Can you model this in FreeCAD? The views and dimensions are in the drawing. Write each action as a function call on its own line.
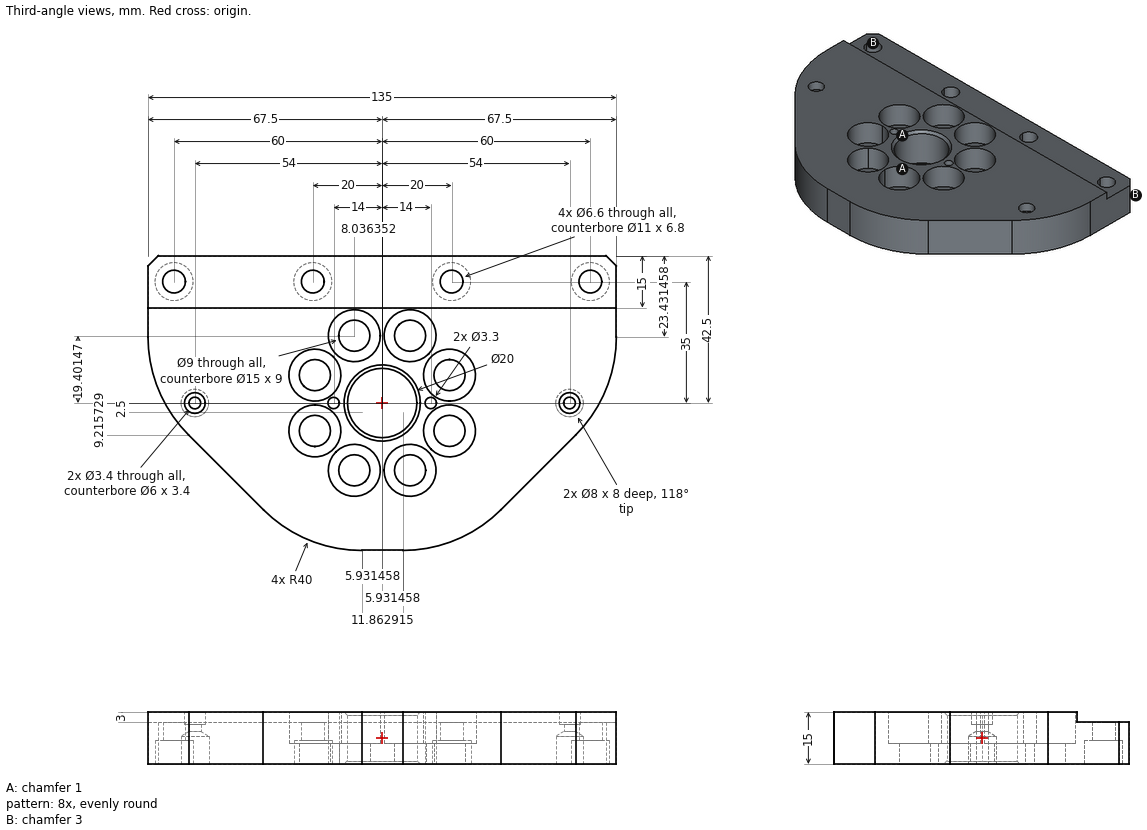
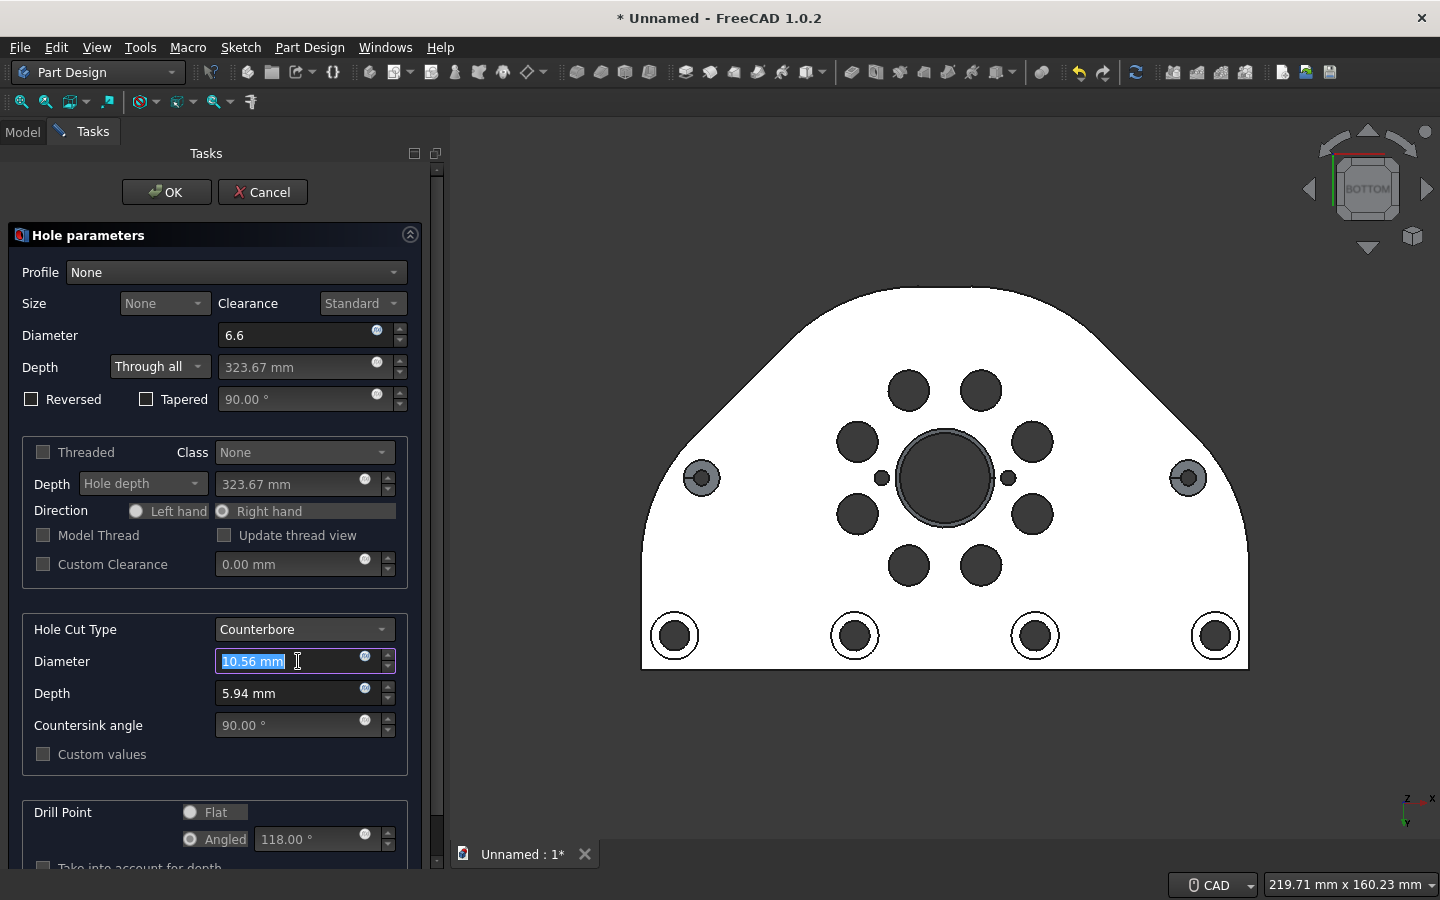
text(11)
key(Tab)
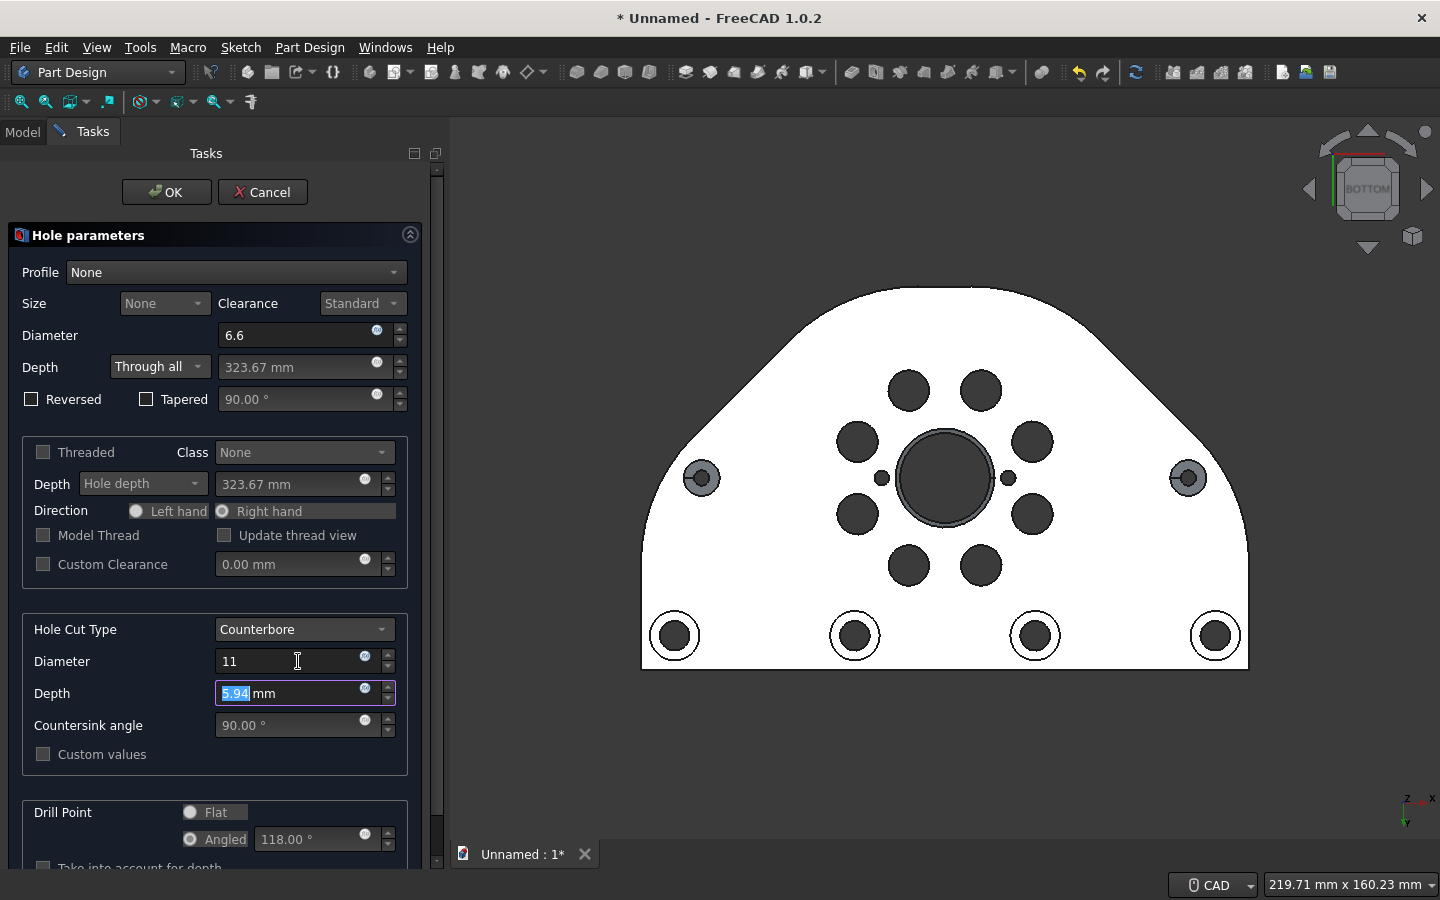
text(6.8)
key(Tab)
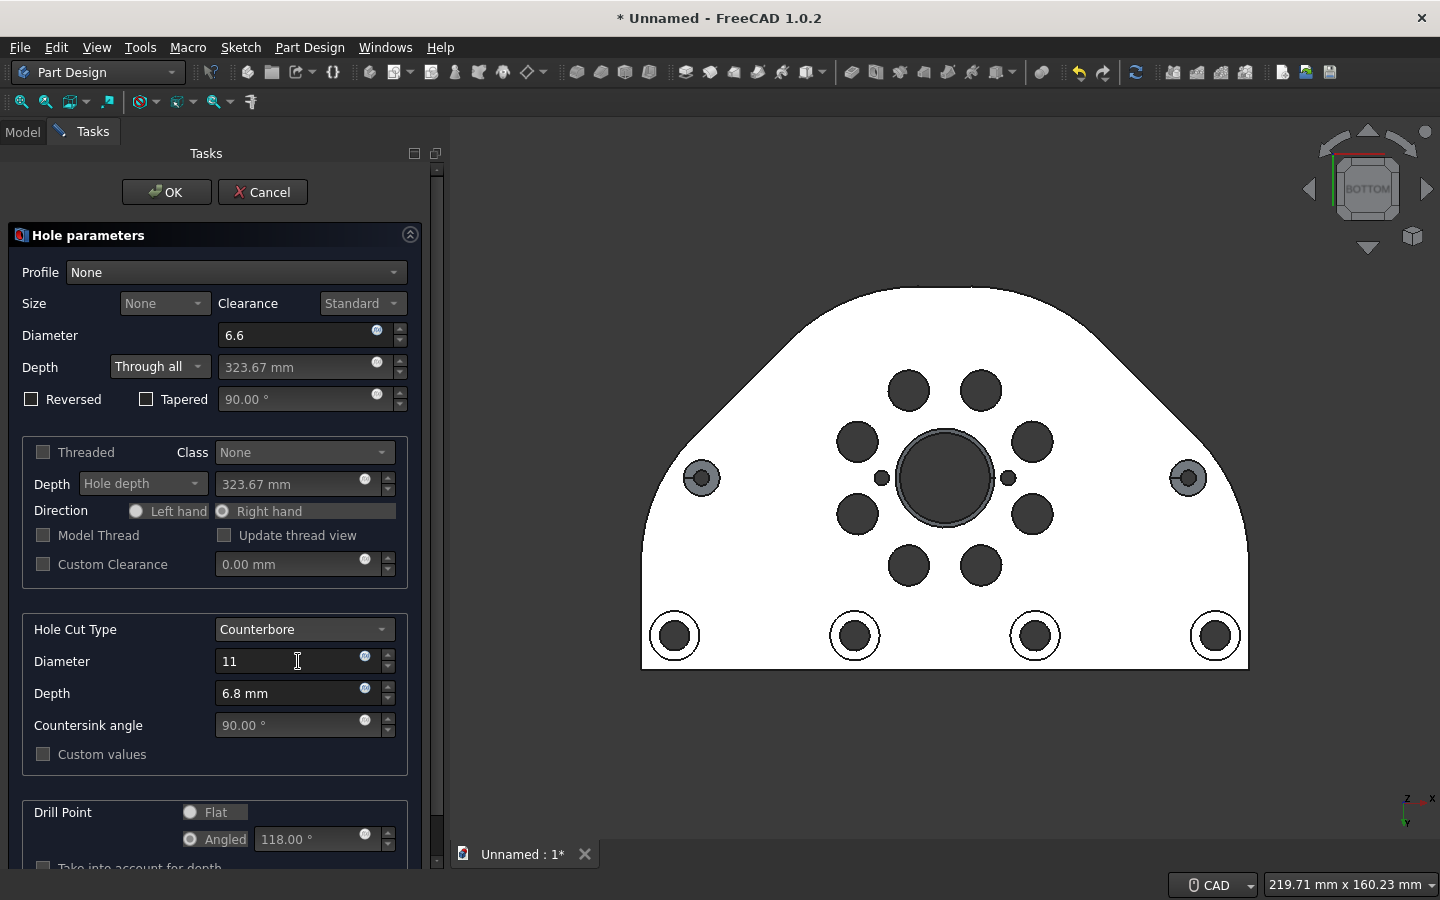
click(167, 192)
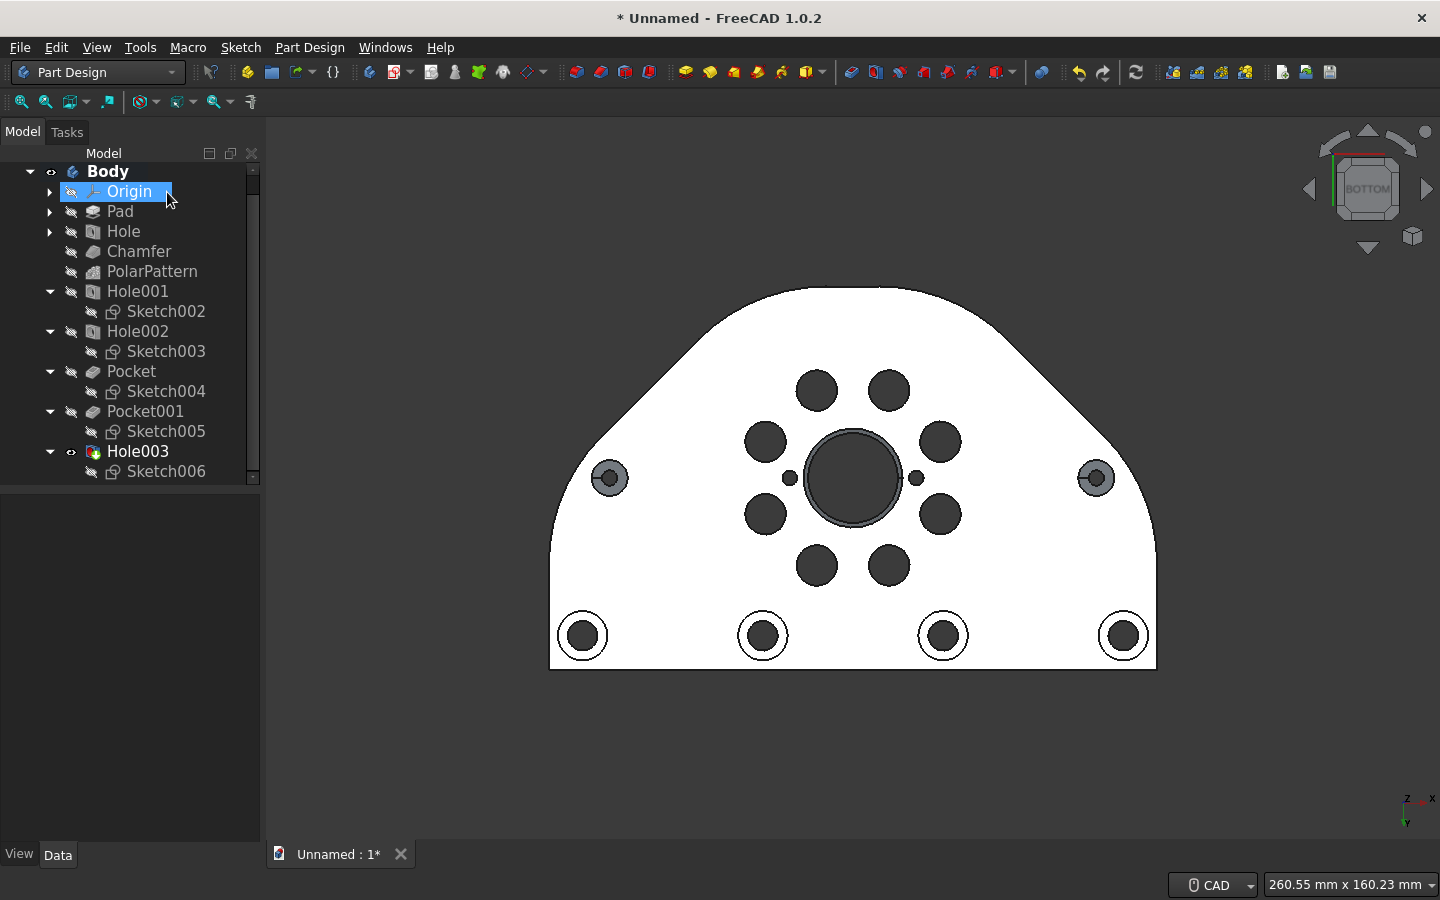
key(0)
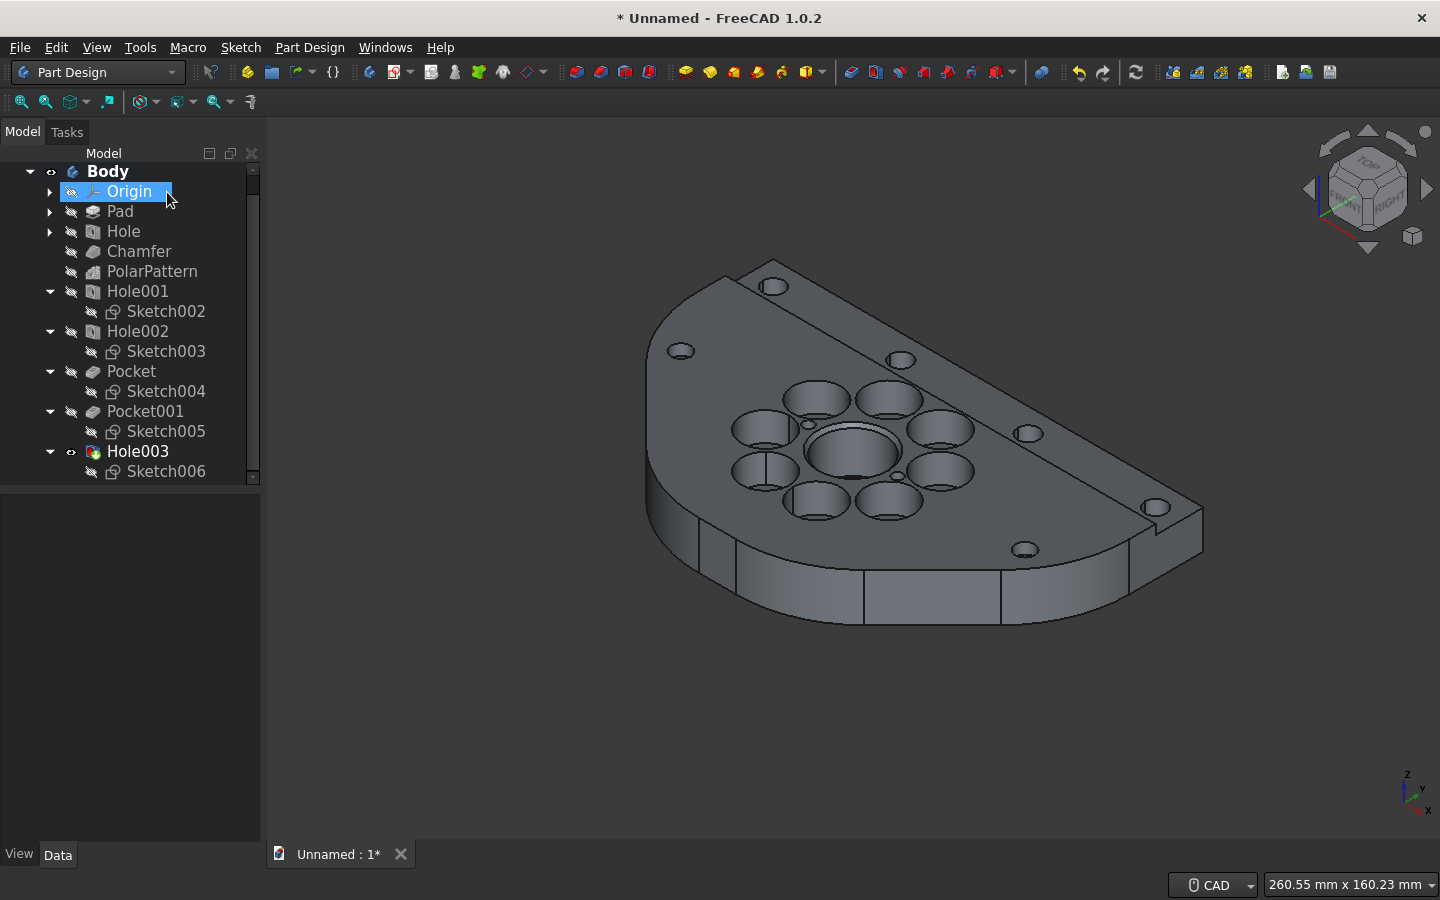
key(2)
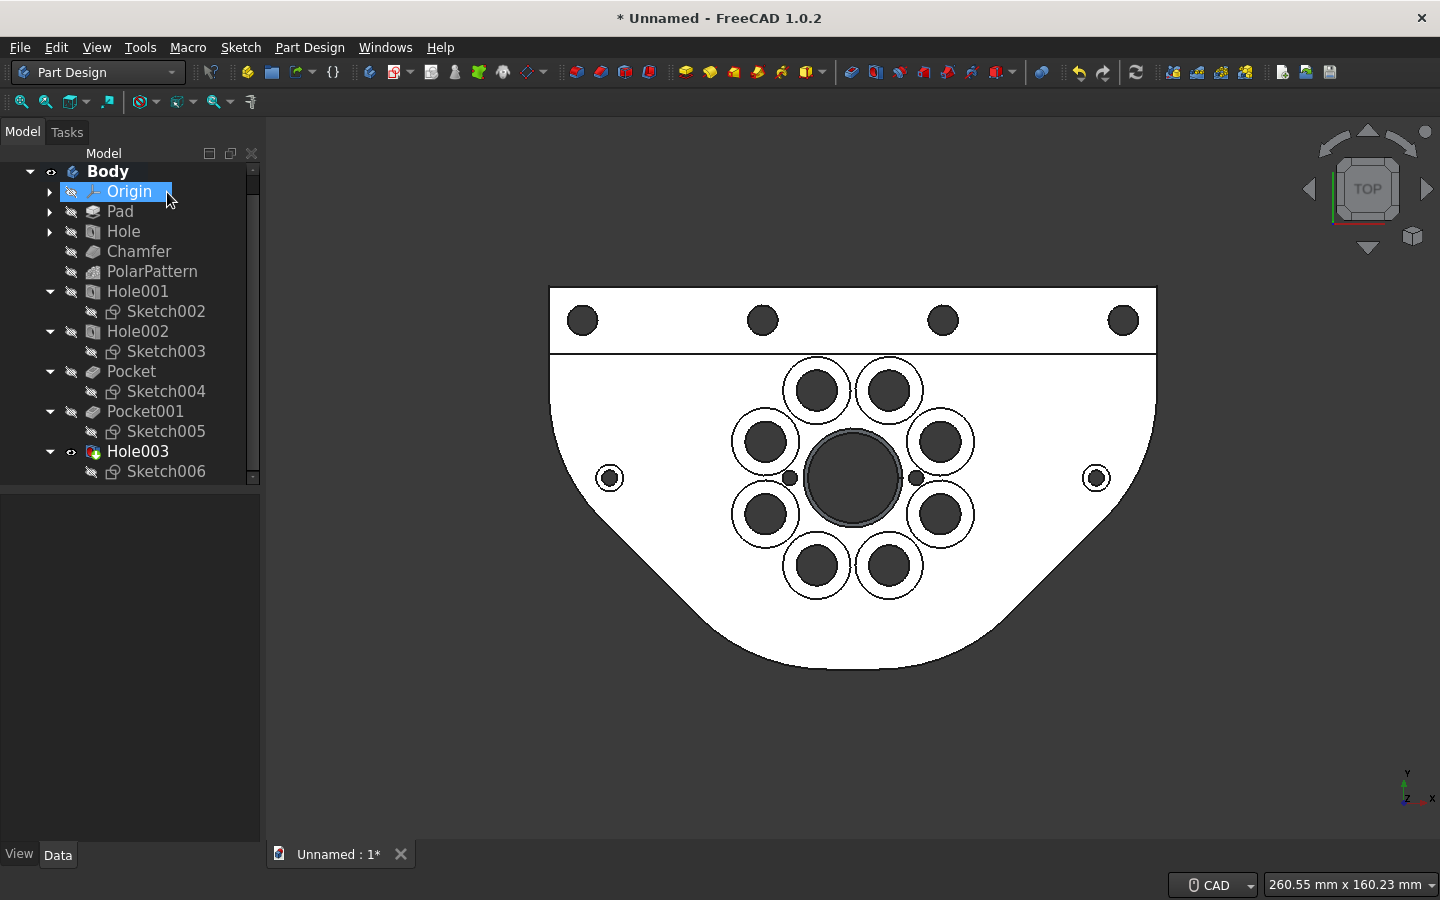
key(1)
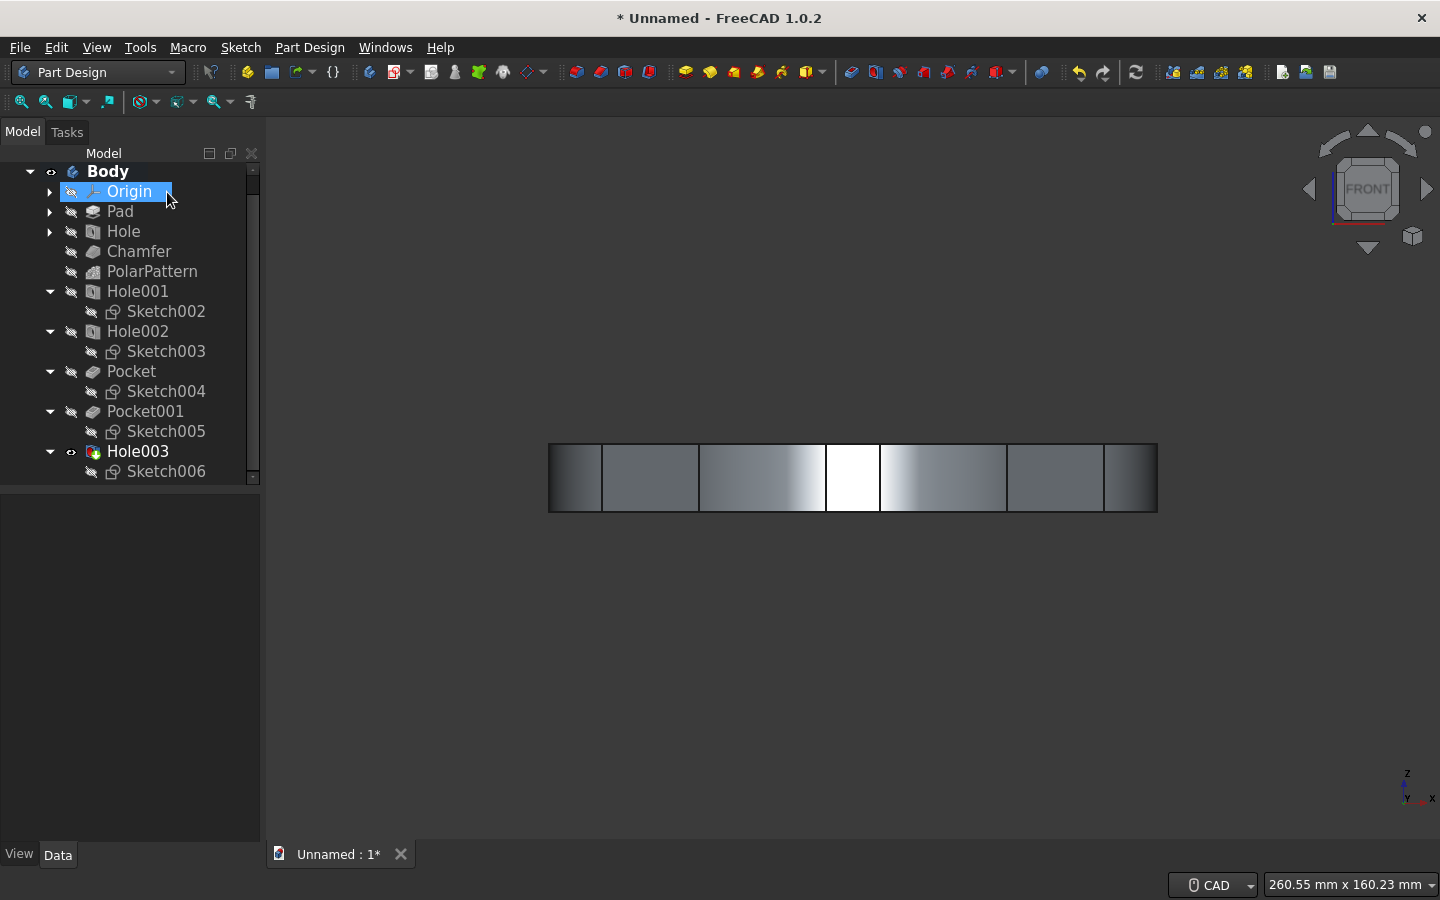
key(3)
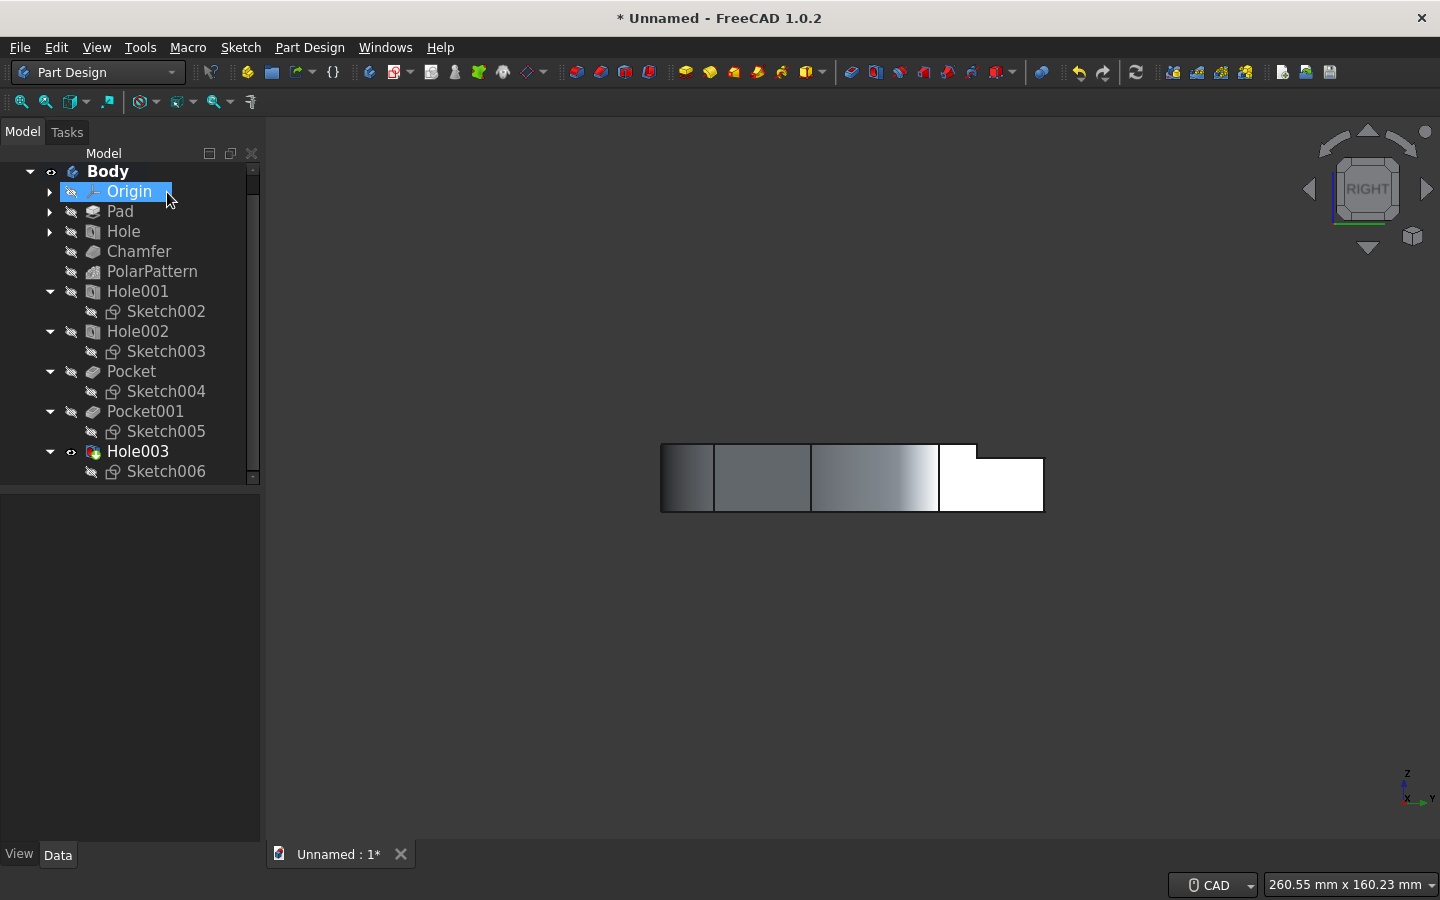
click(22, 102)